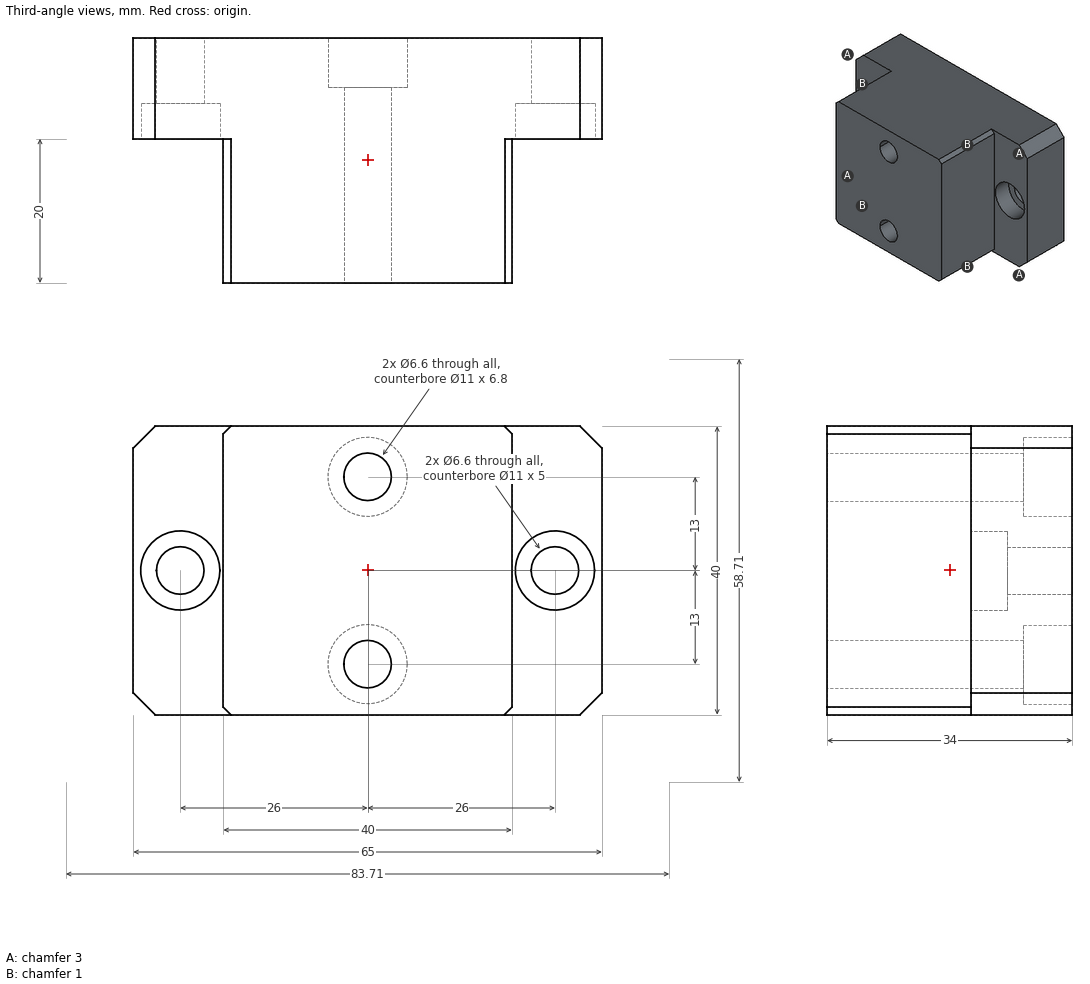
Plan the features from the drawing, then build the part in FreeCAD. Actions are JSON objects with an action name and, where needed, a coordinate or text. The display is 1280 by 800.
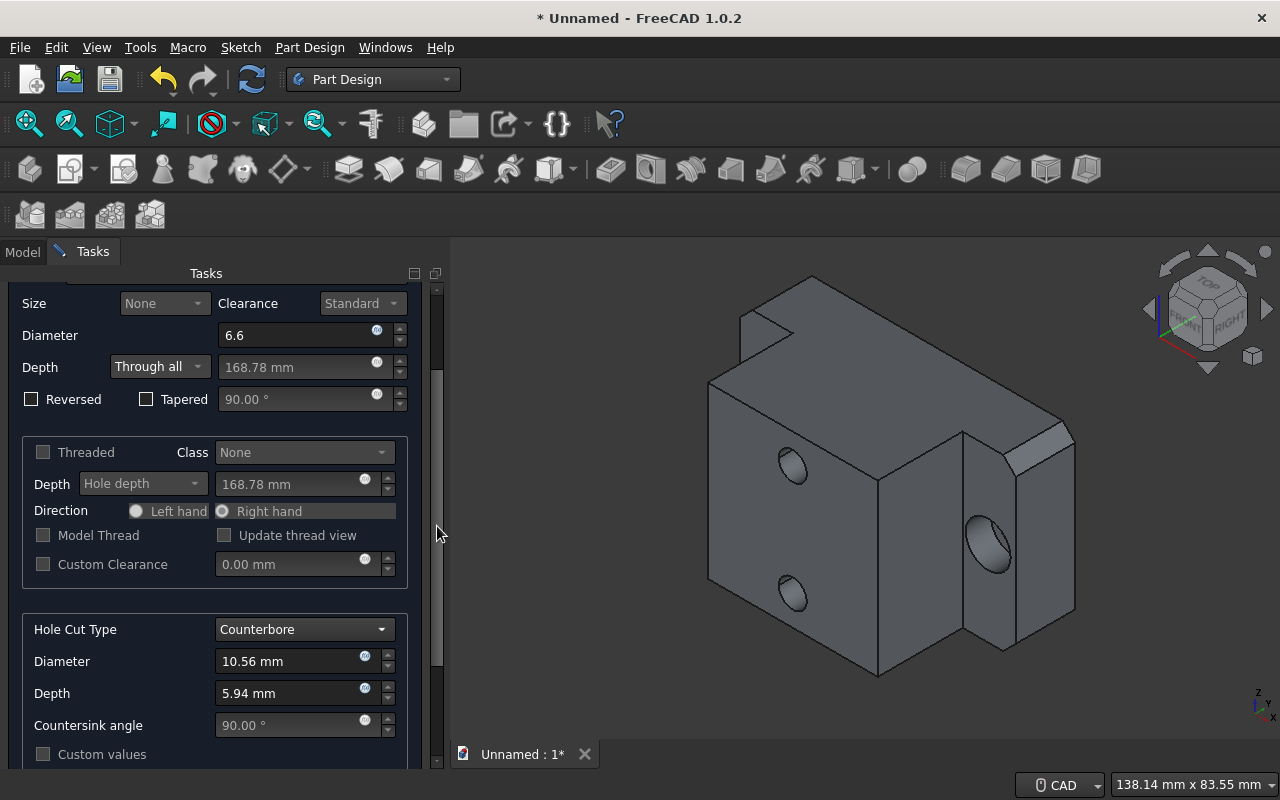
{"action": "triple_click", "coordinate": [298, 661]}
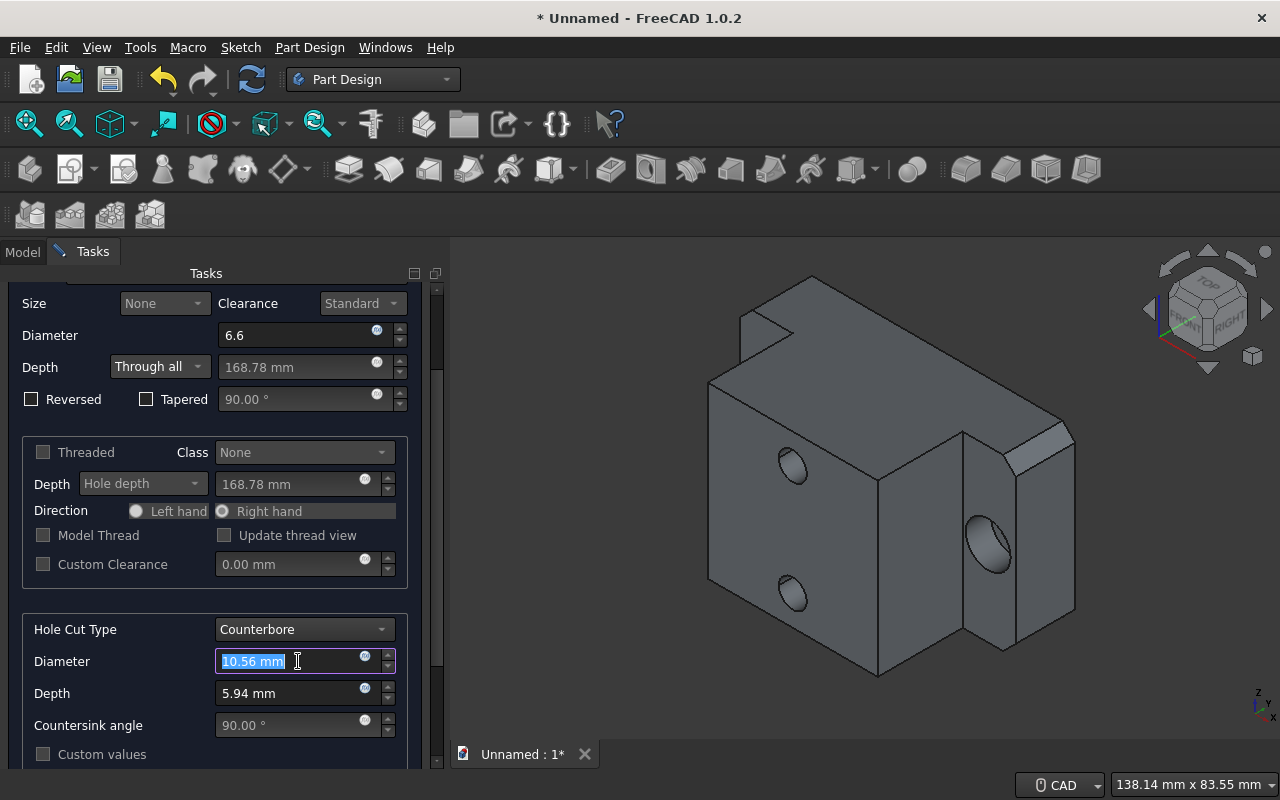
{"action": "type", "text": "11"}
{"action": "key", "text": "Tab"}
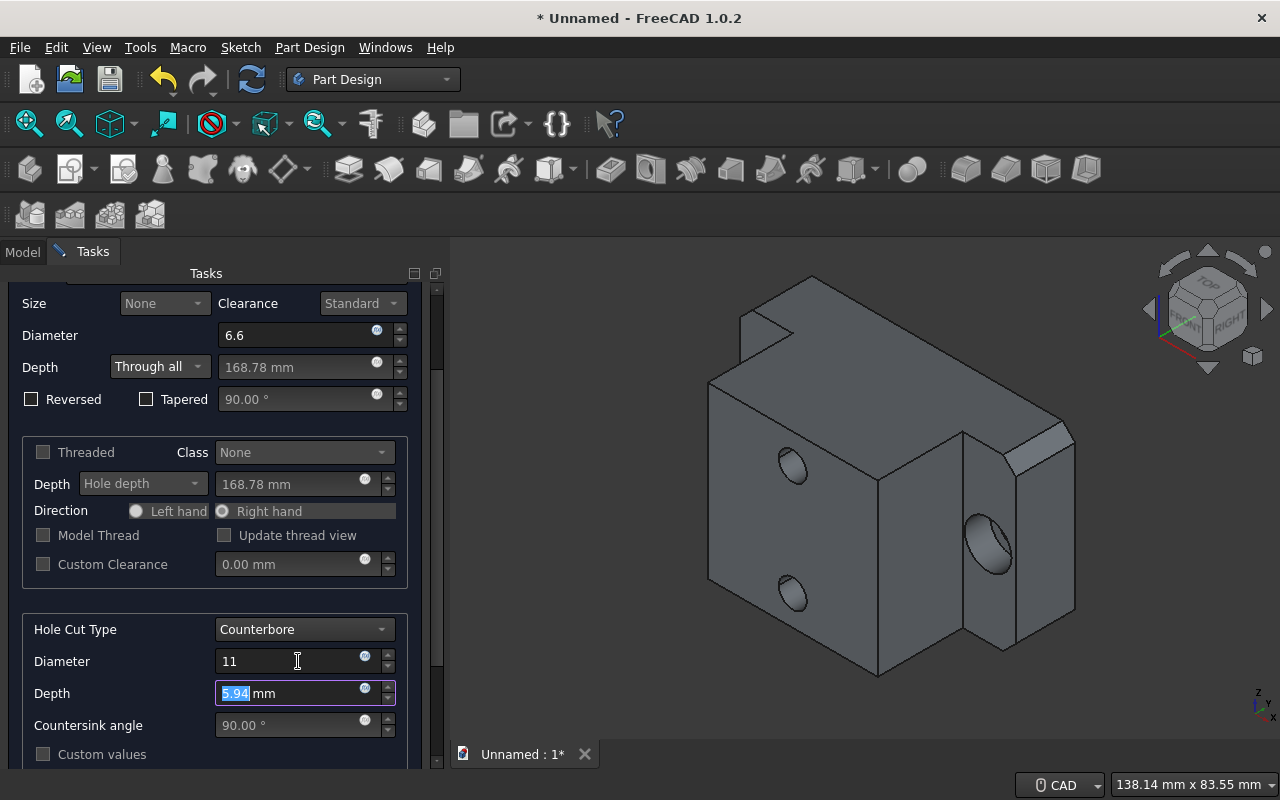
{"action": "type", "text": "5"}
{"action": "key", "text": "Tab"}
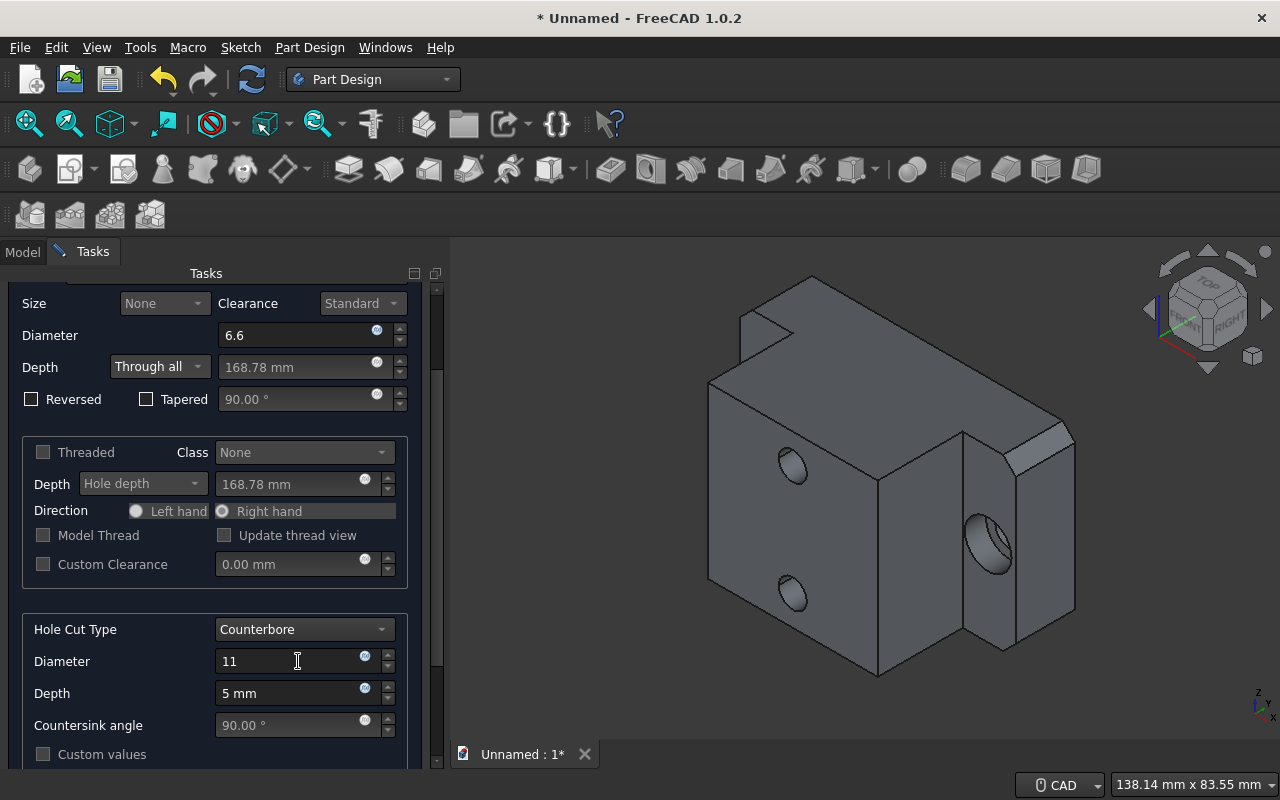
{"action": "scroll", "coordinate": [437, 526], "scroll_direction": "up", "scroll_amount": 3}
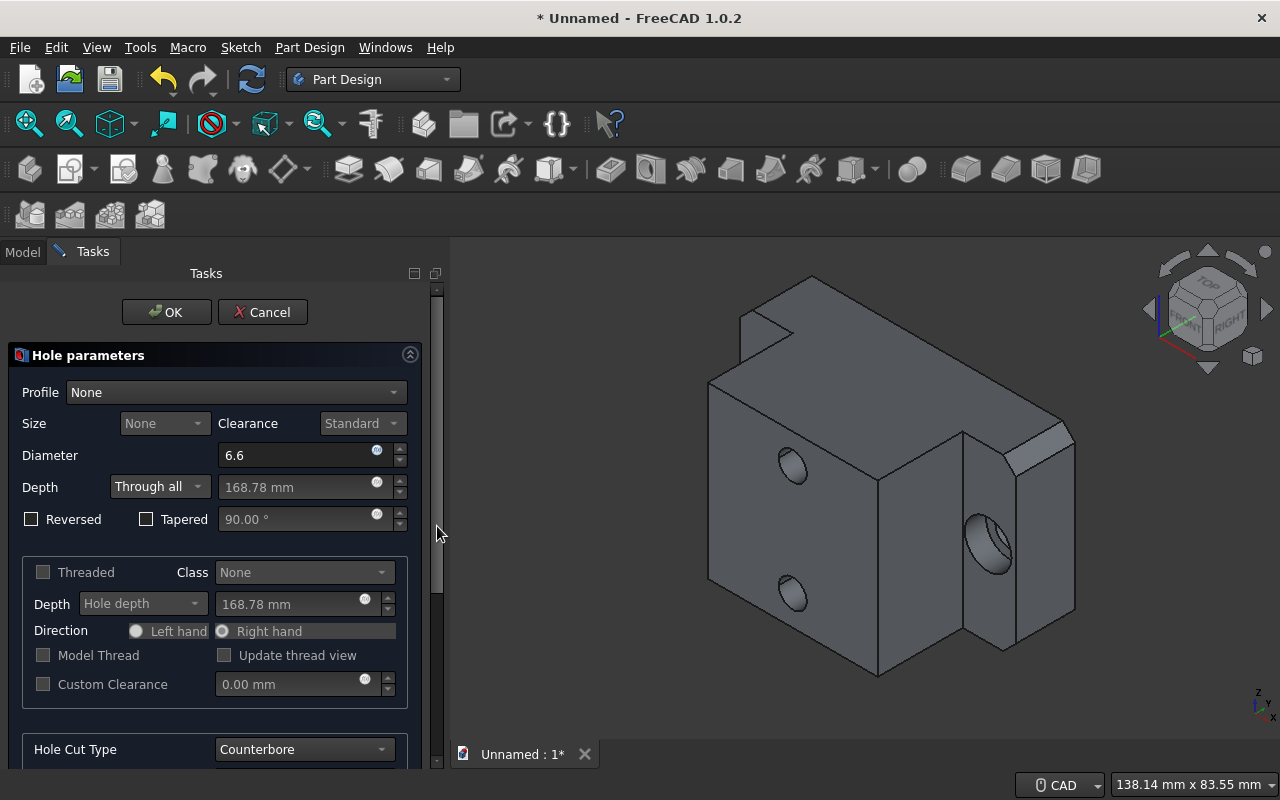
{"action": "left_click", "coordinate": [167, 312]}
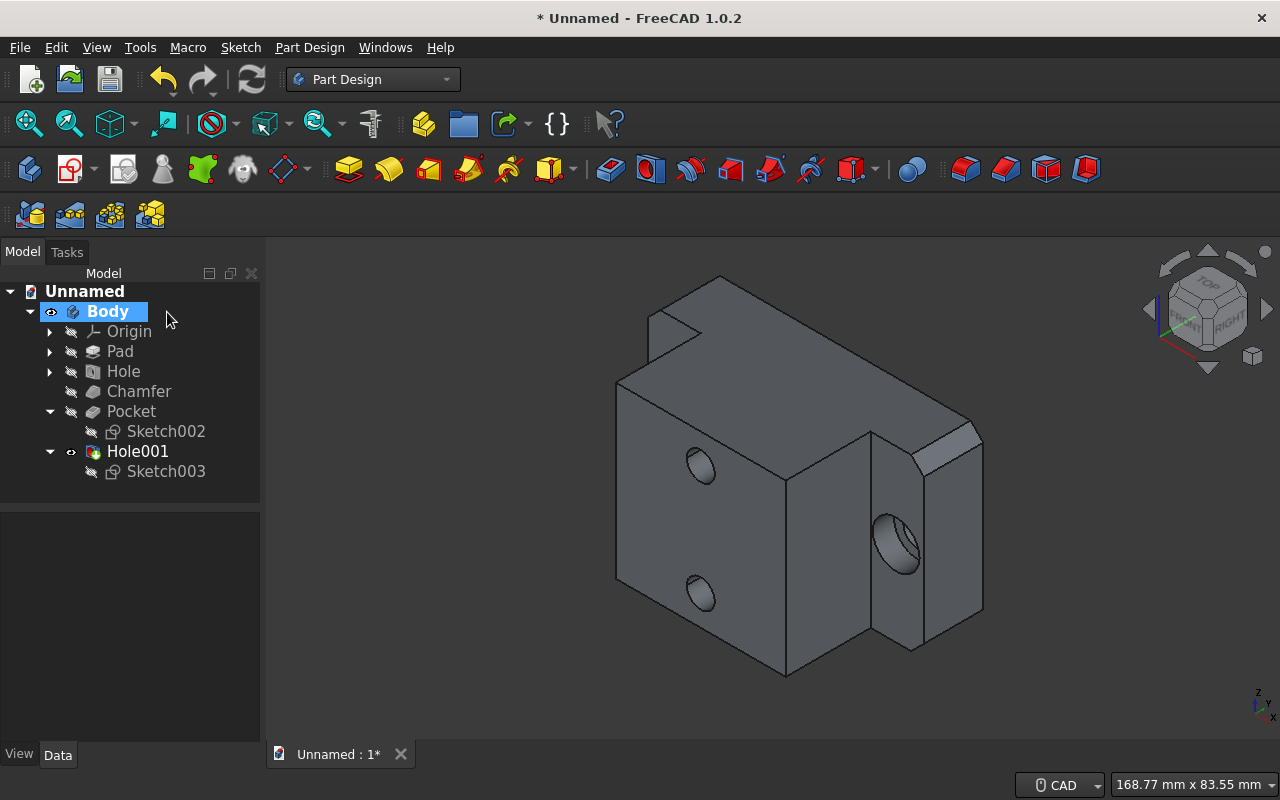
{"action": "left_click", "coordinate": [828, 455]}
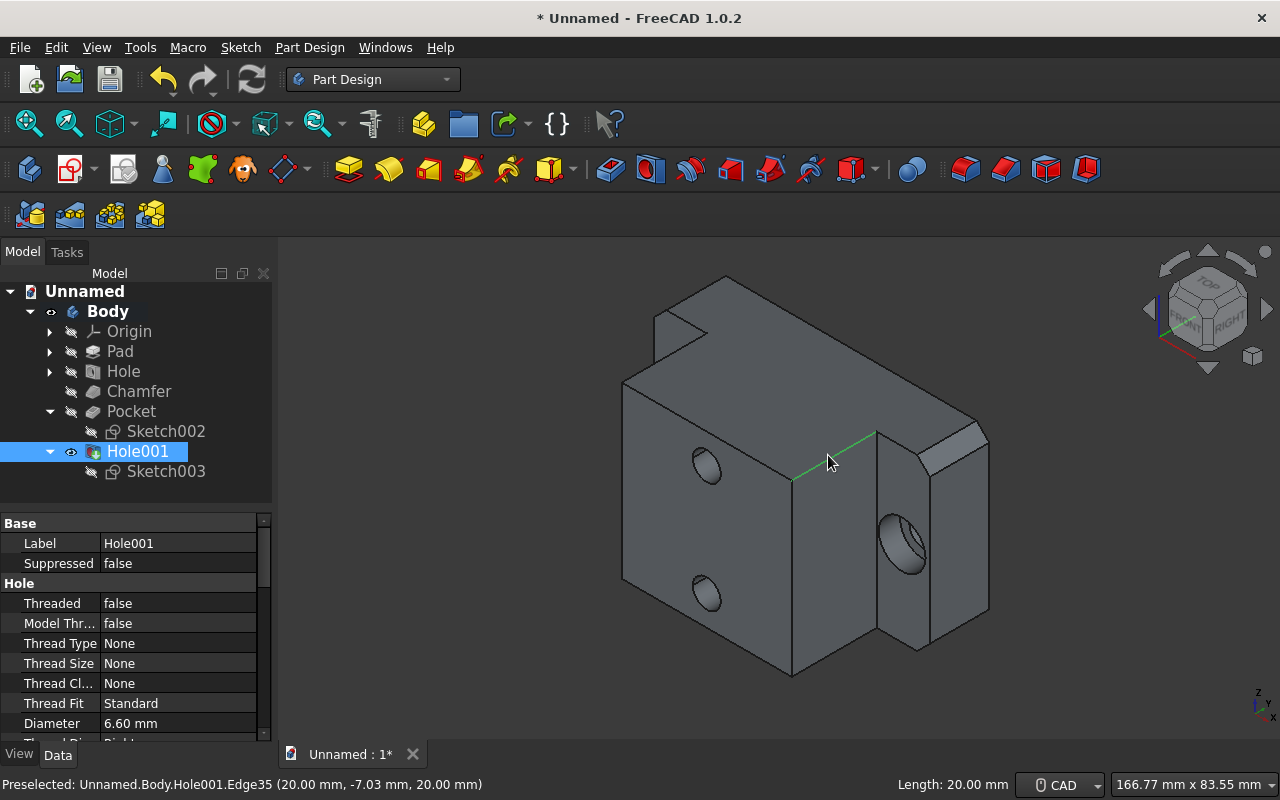
{"action": "key", "text": "2"}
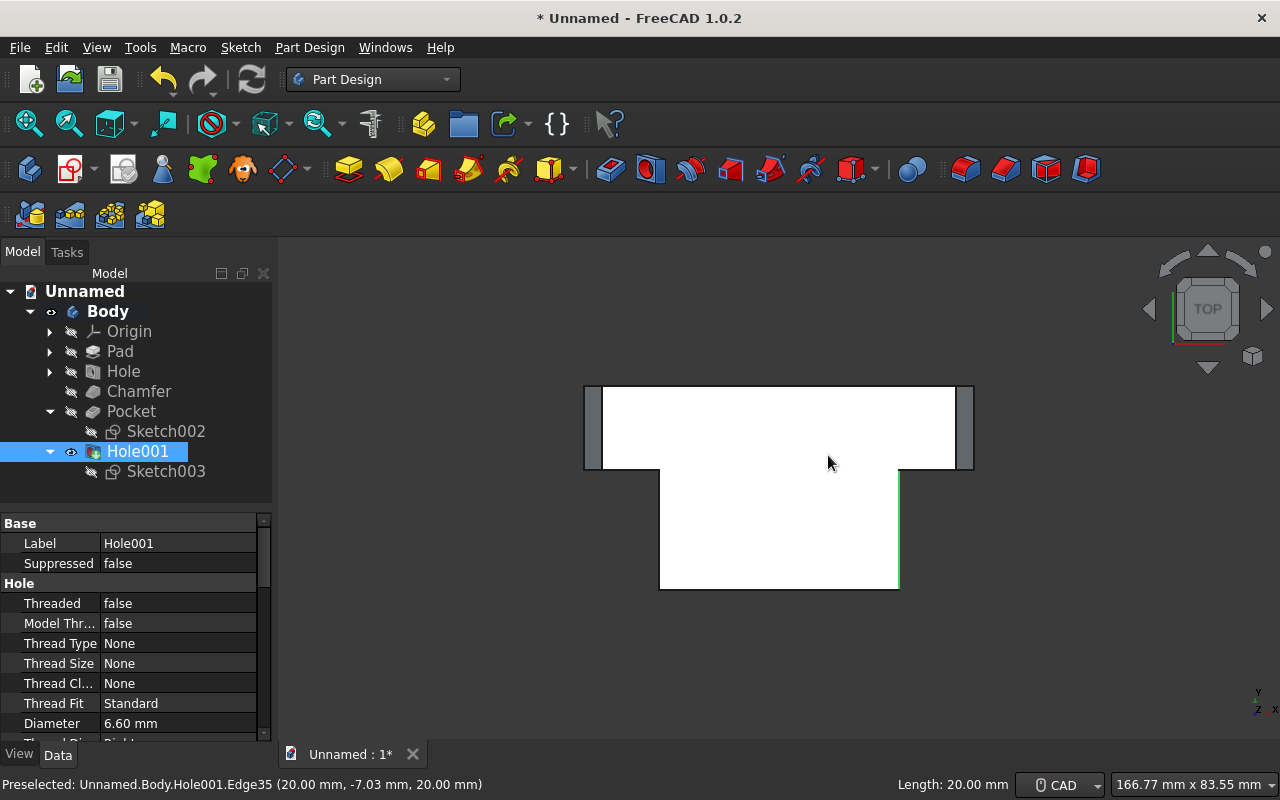
{"action": "key", "text": "v f"}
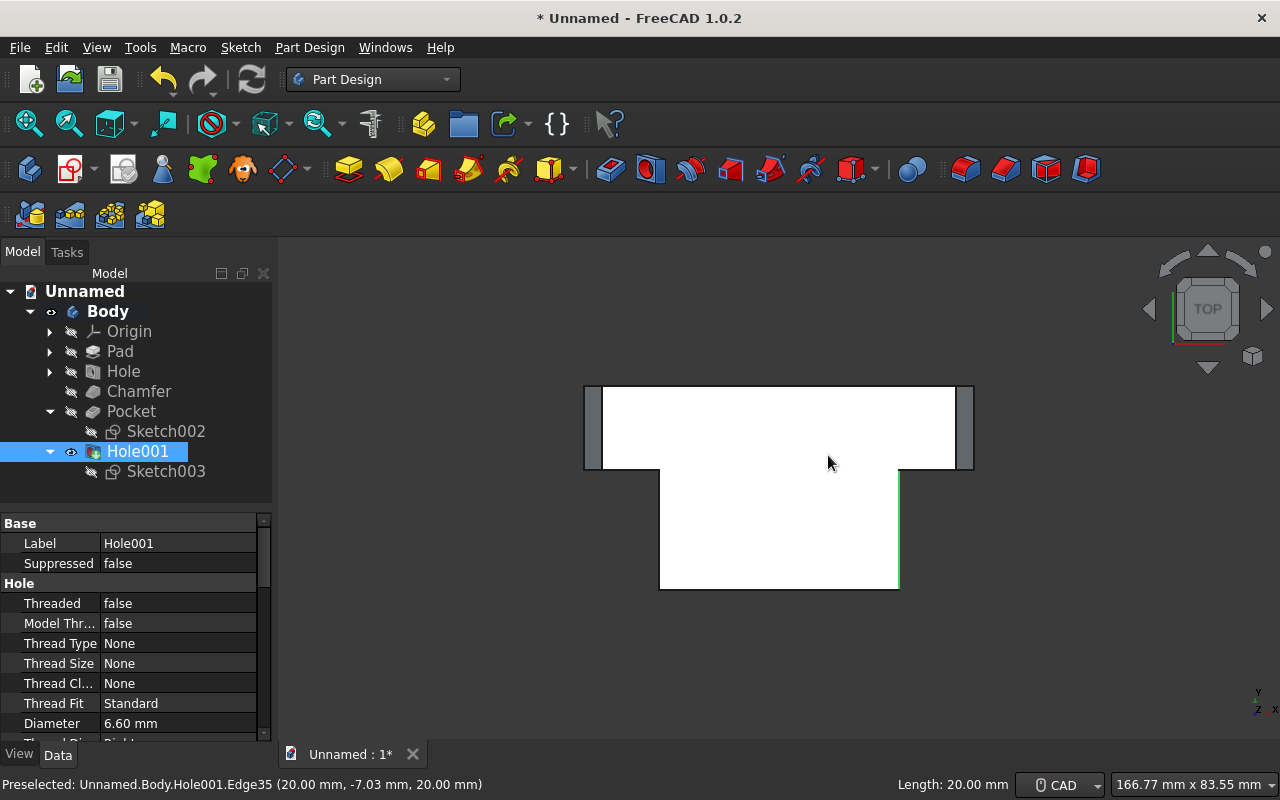
{"action": "left_click", "coordinate": [659, 529], "text": "ctrl"}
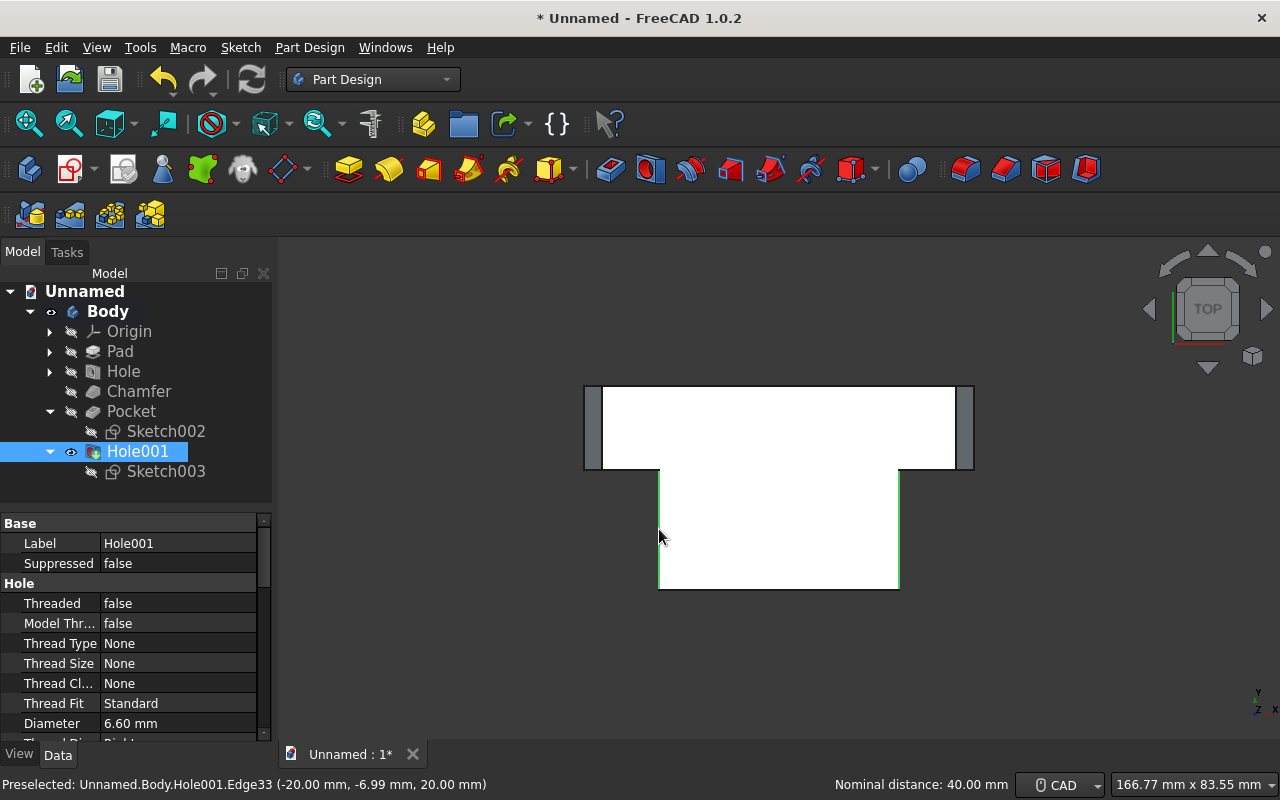
{"action": "key", "text": "0"}